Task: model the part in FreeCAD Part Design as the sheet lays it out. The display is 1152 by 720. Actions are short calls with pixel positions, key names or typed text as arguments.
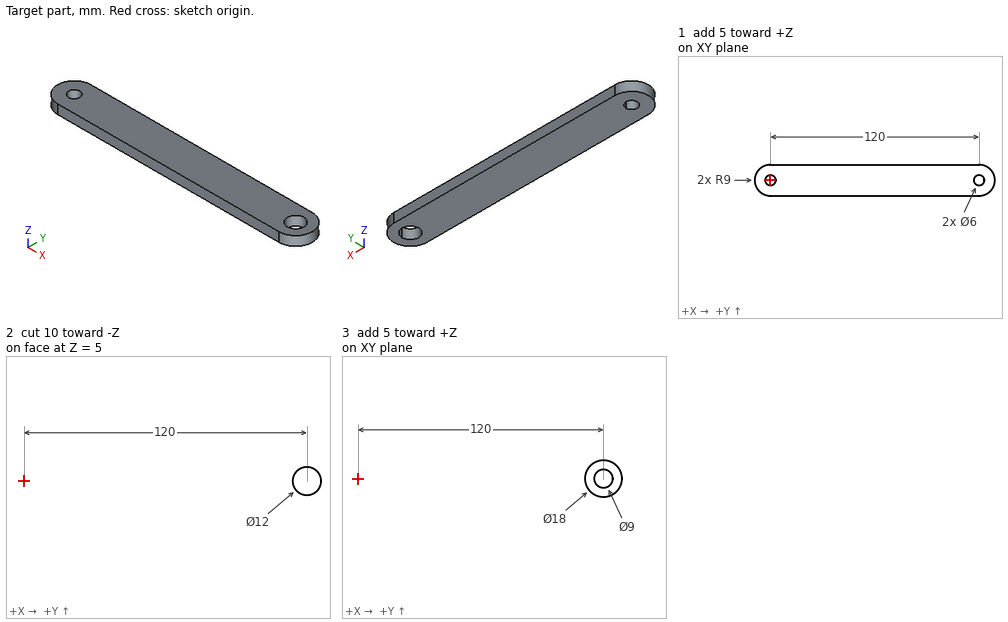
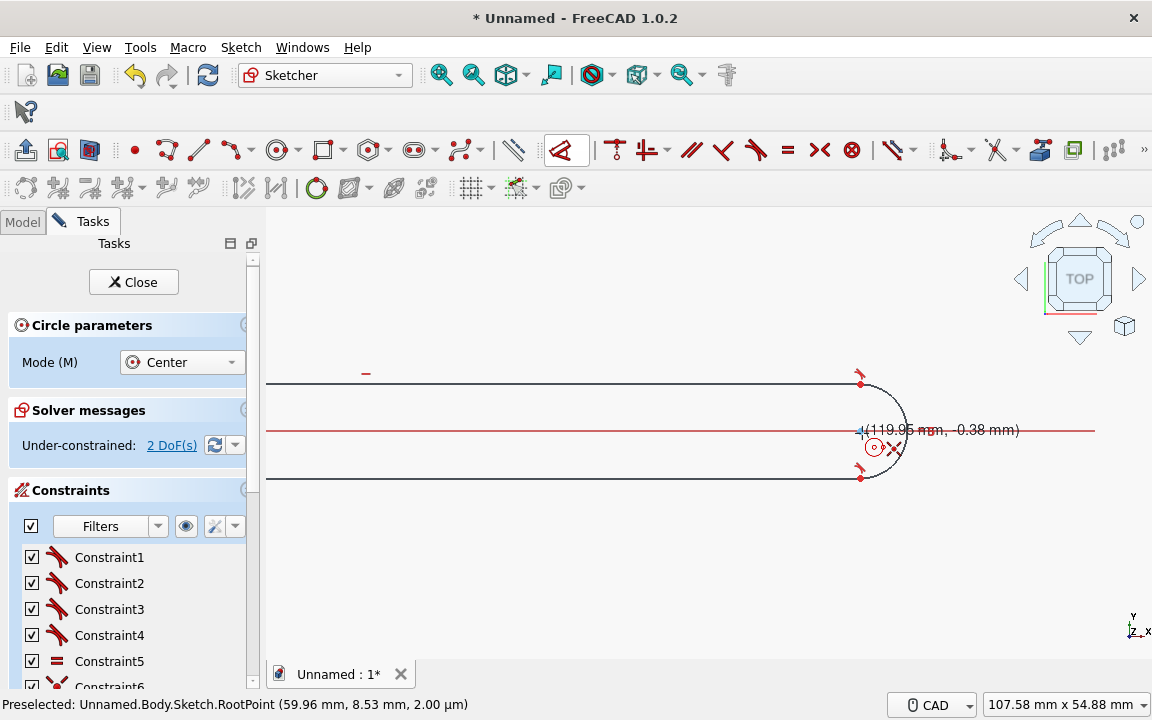
click(861, 412)
move(879, 414)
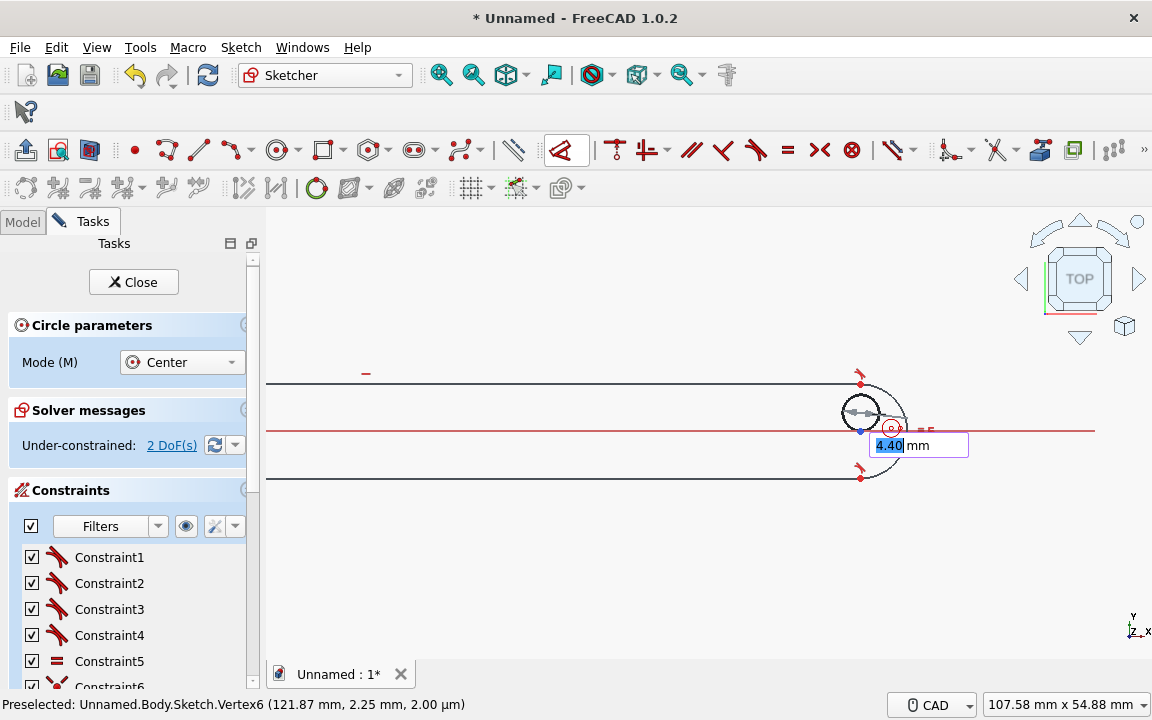
text(6)
key(Return)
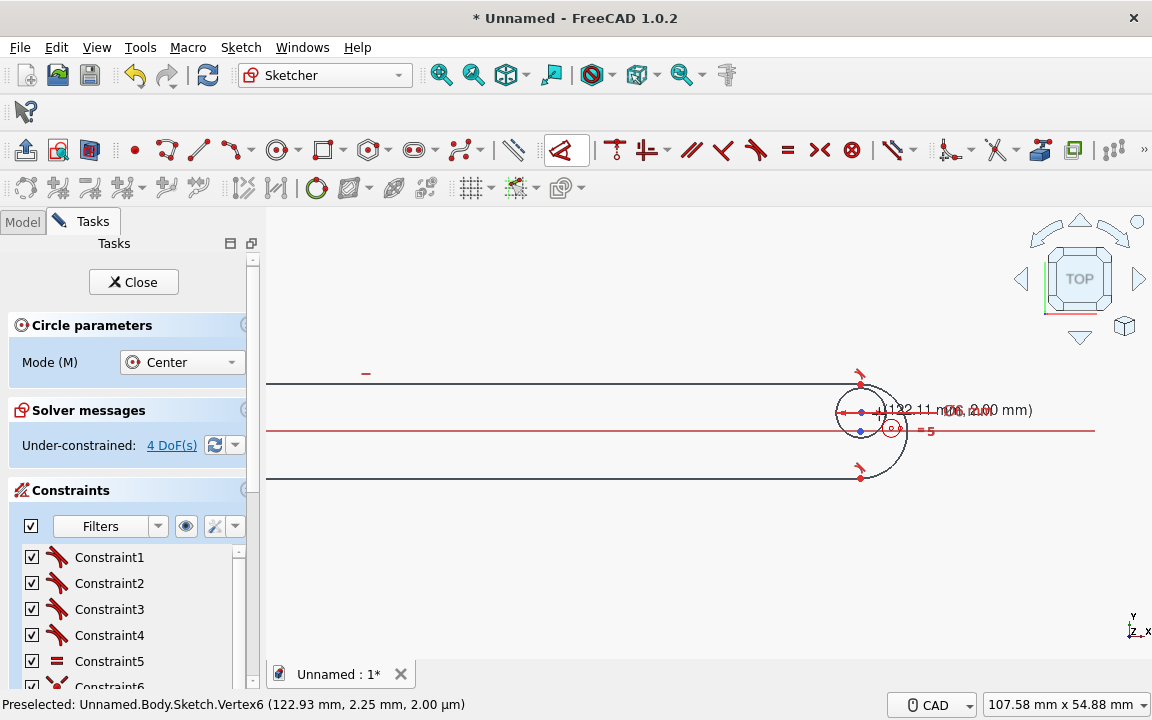
scroll(863, 434, down, 4)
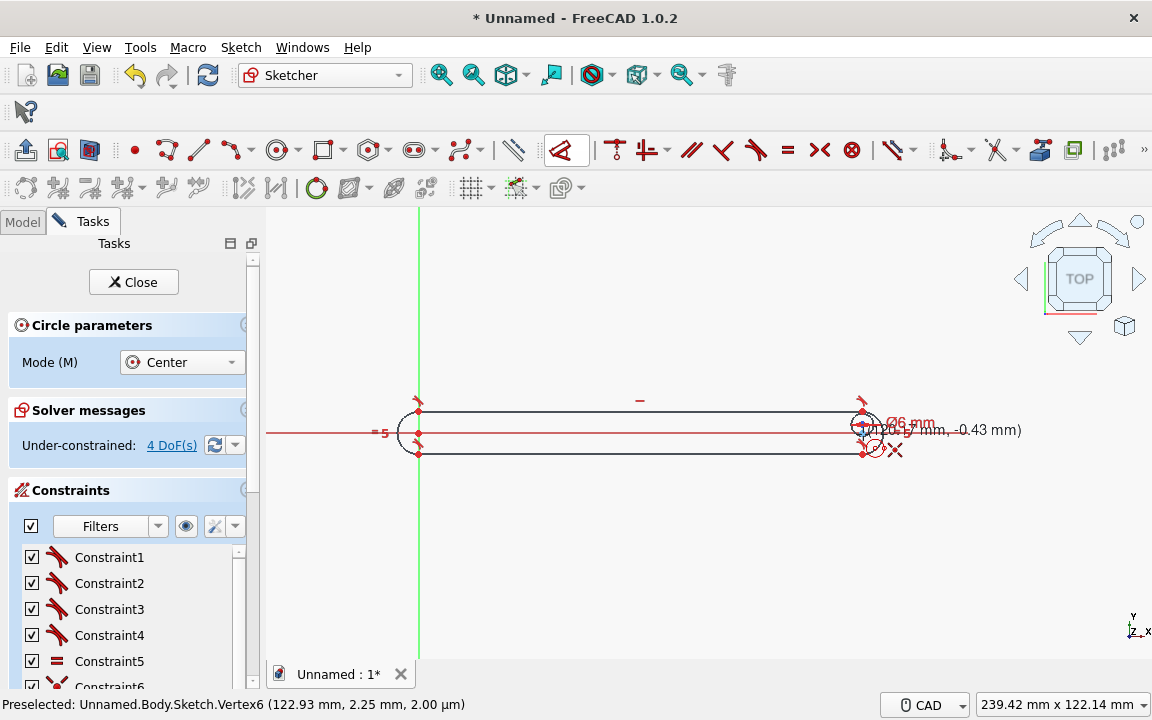
scroll(419, 433, up, 4)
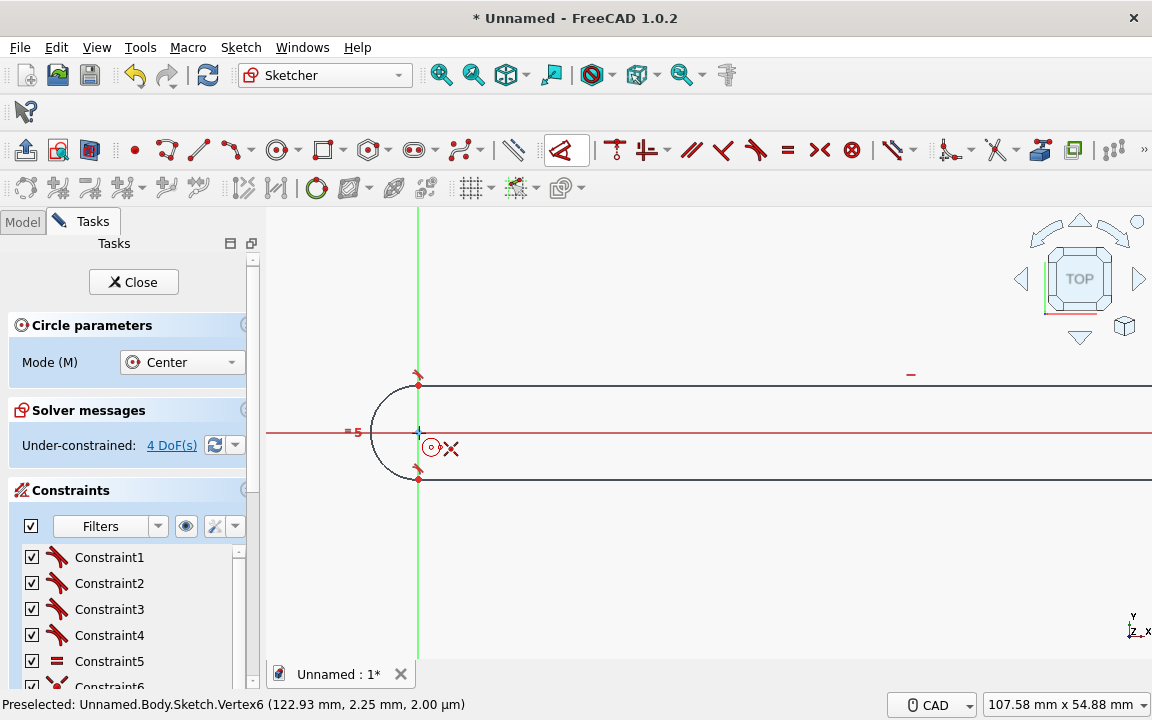
click(418, 433)
move(436, 415)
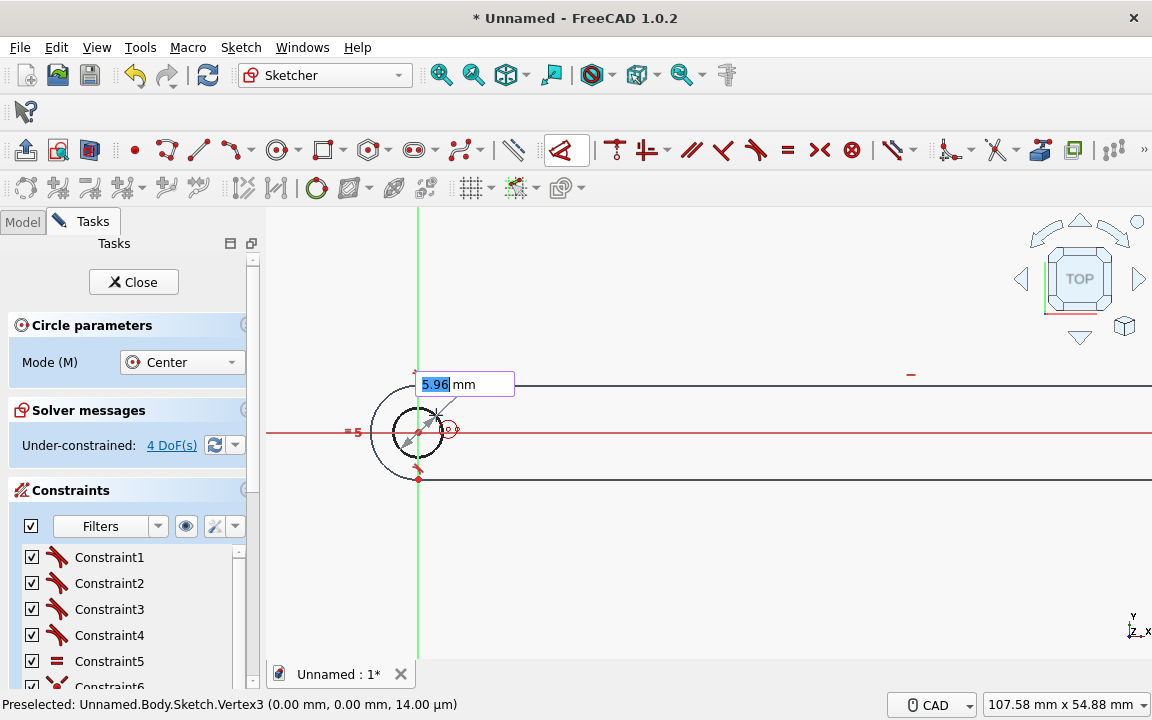
text(6)
key(Return)
key(Escape)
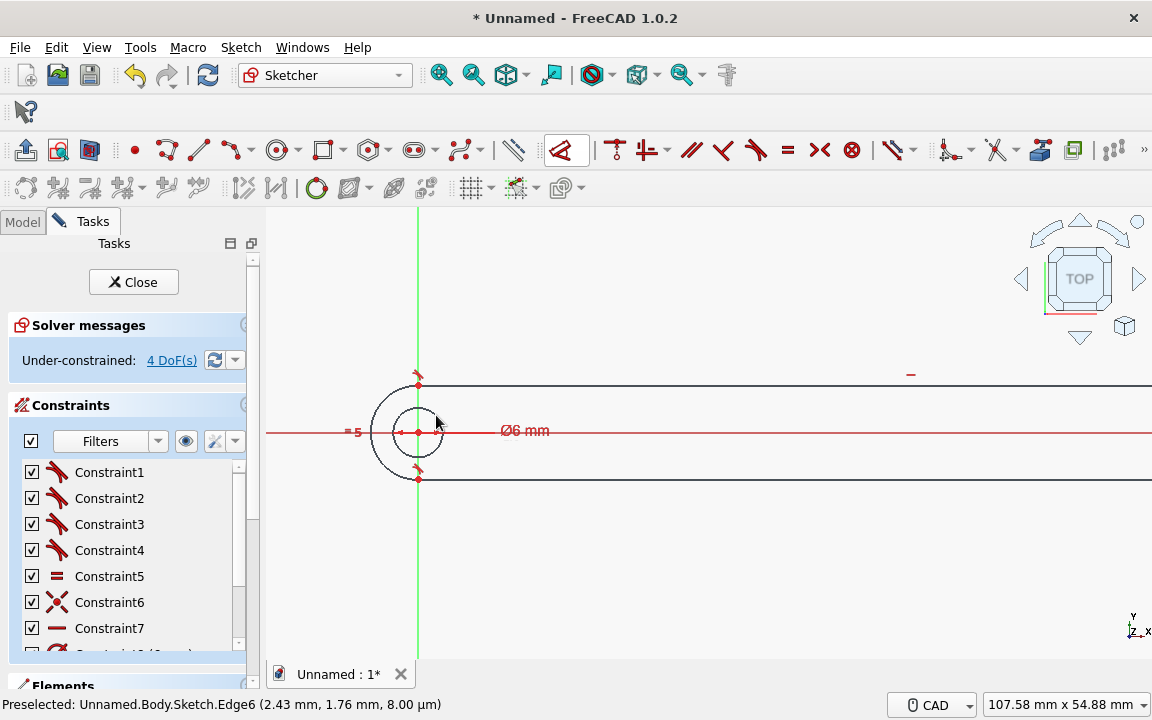
scroll(419, 433, down, 4)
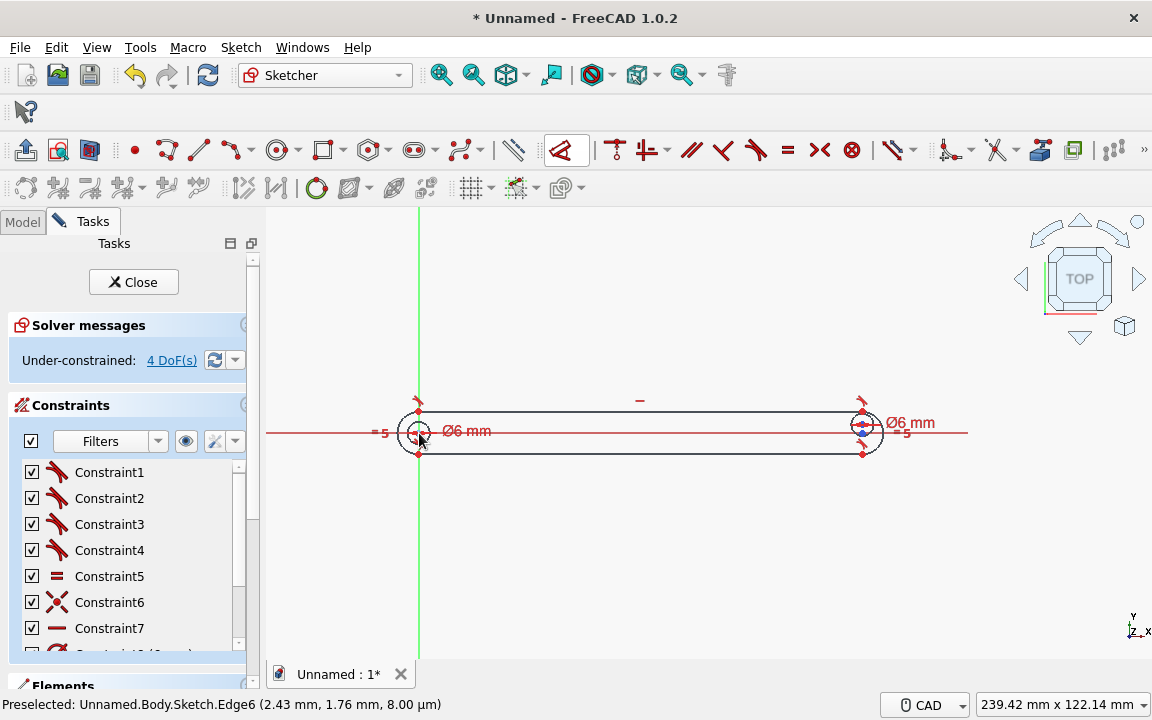
scroll(855, 417, up, 6)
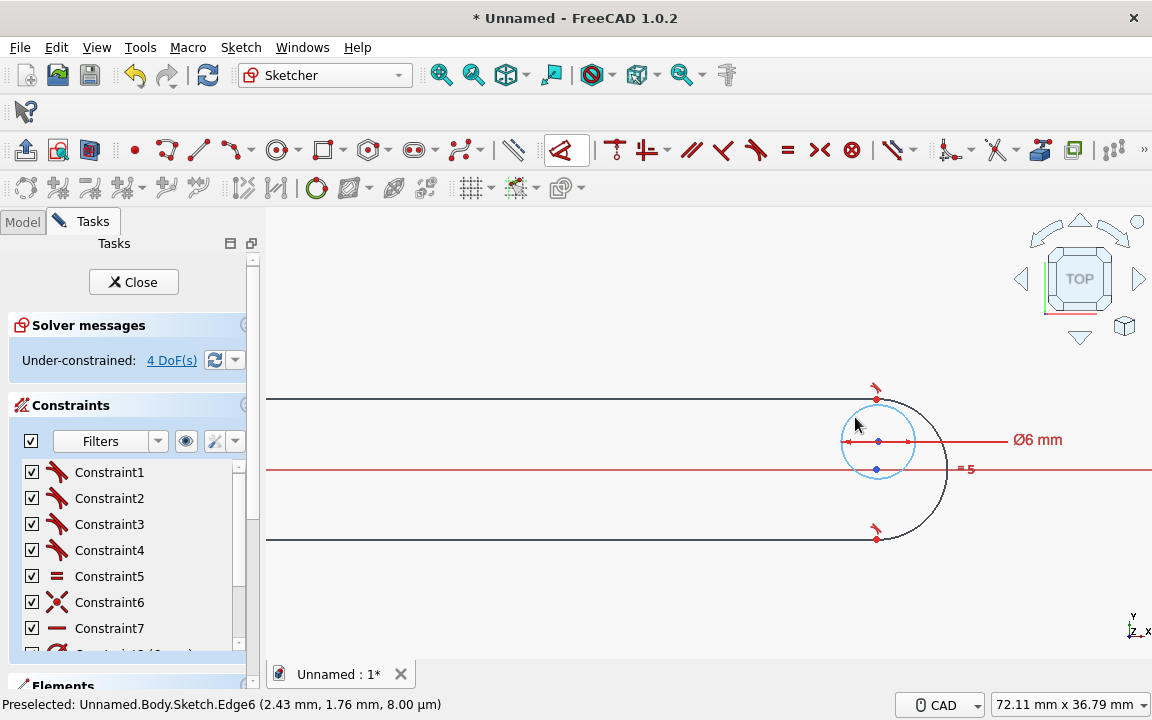
click(852, 416)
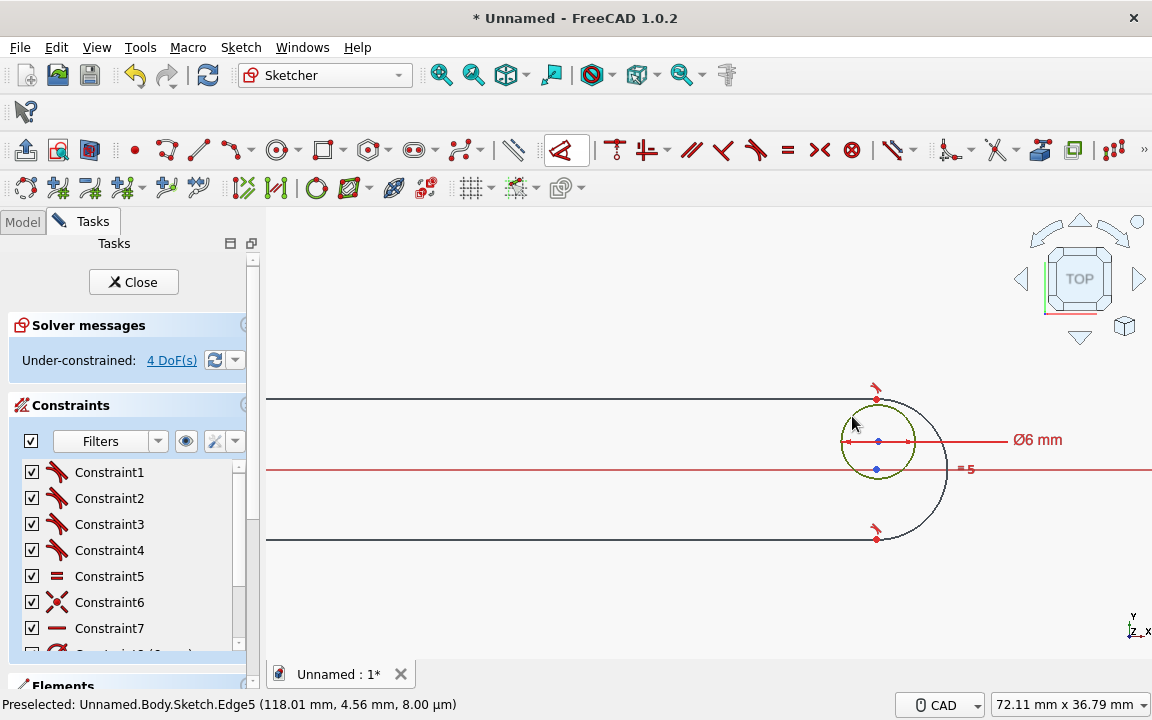
click(934, 511)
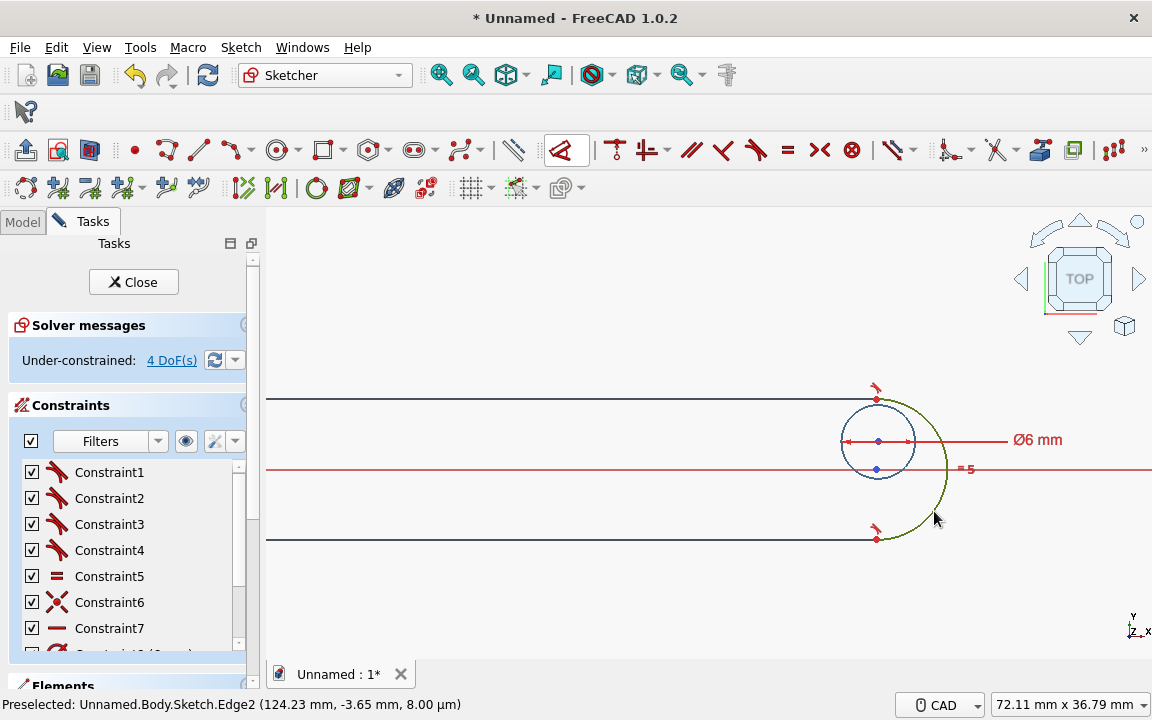
click(616, 150)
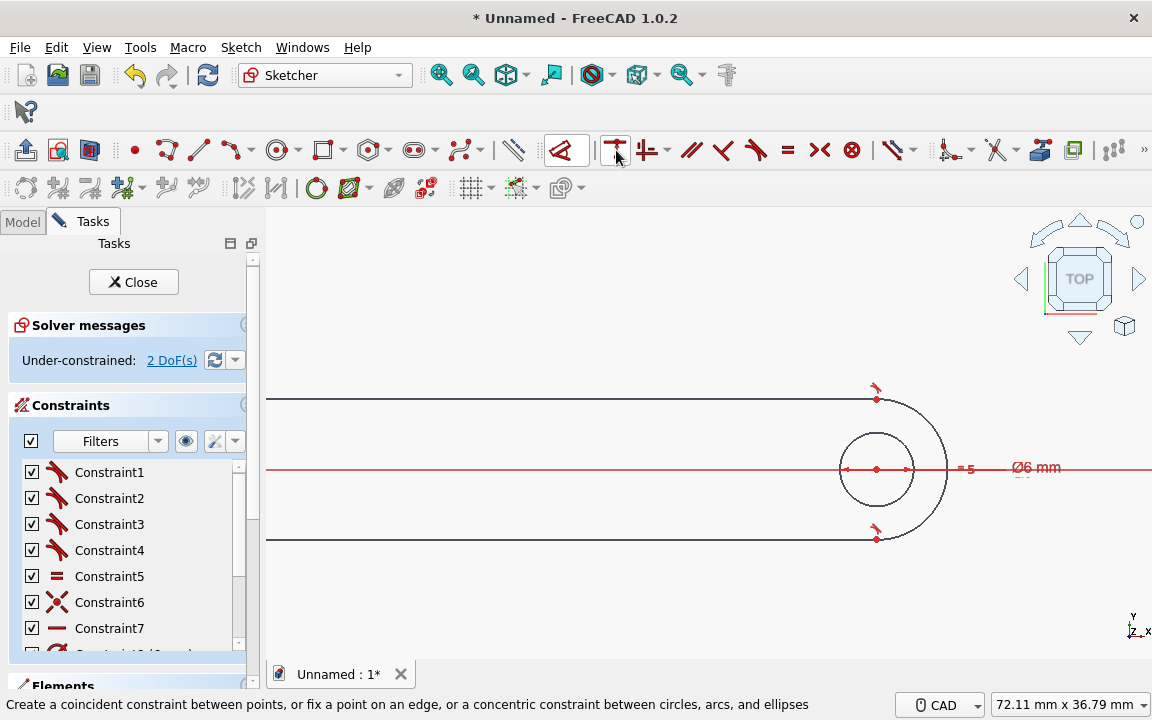
scroll(855, 417, down, 6)